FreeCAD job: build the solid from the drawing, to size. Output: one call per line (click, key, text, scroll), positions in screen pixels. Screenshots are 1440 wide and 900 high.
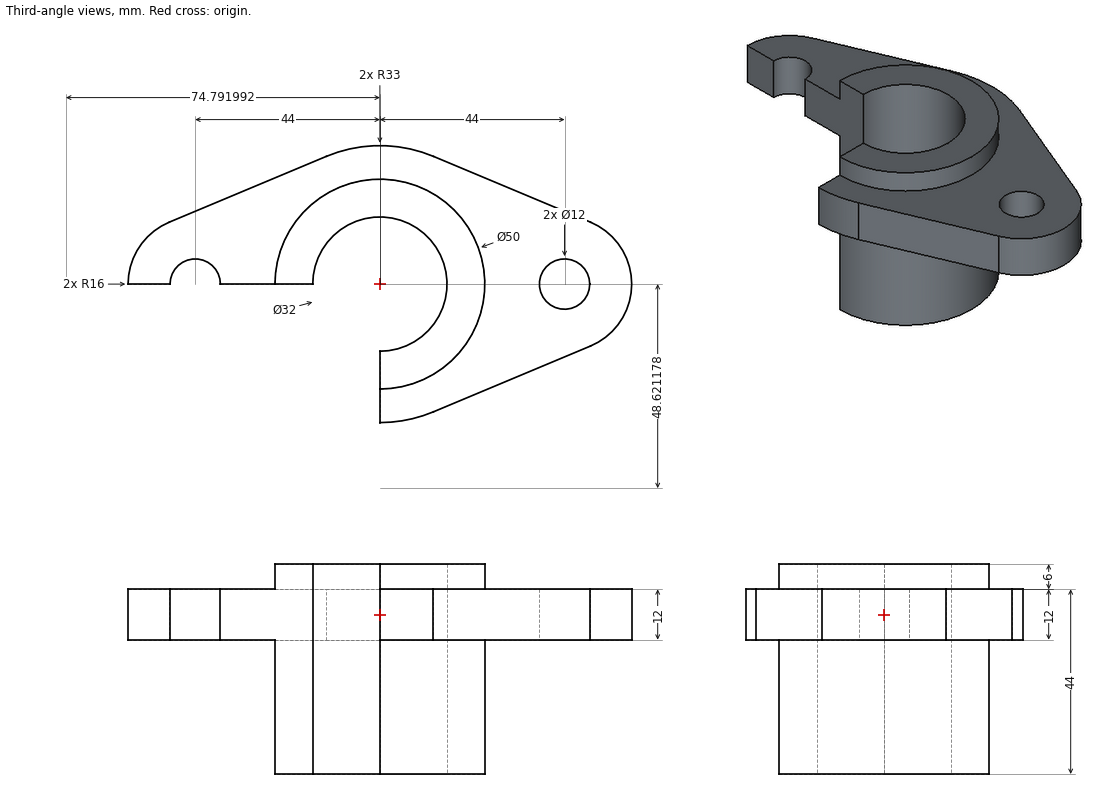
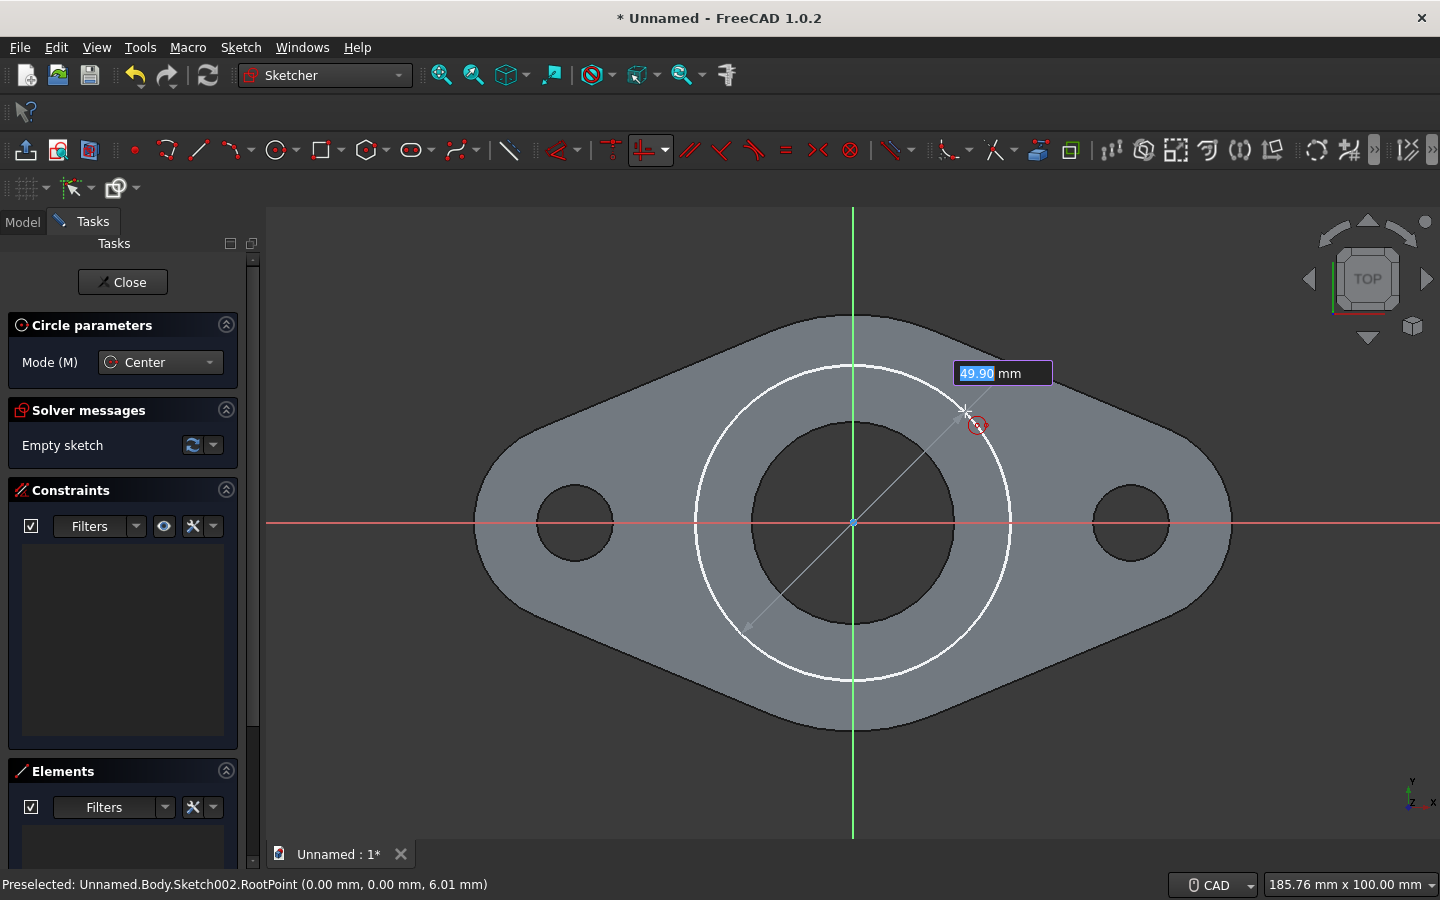
text(50)
key(Return)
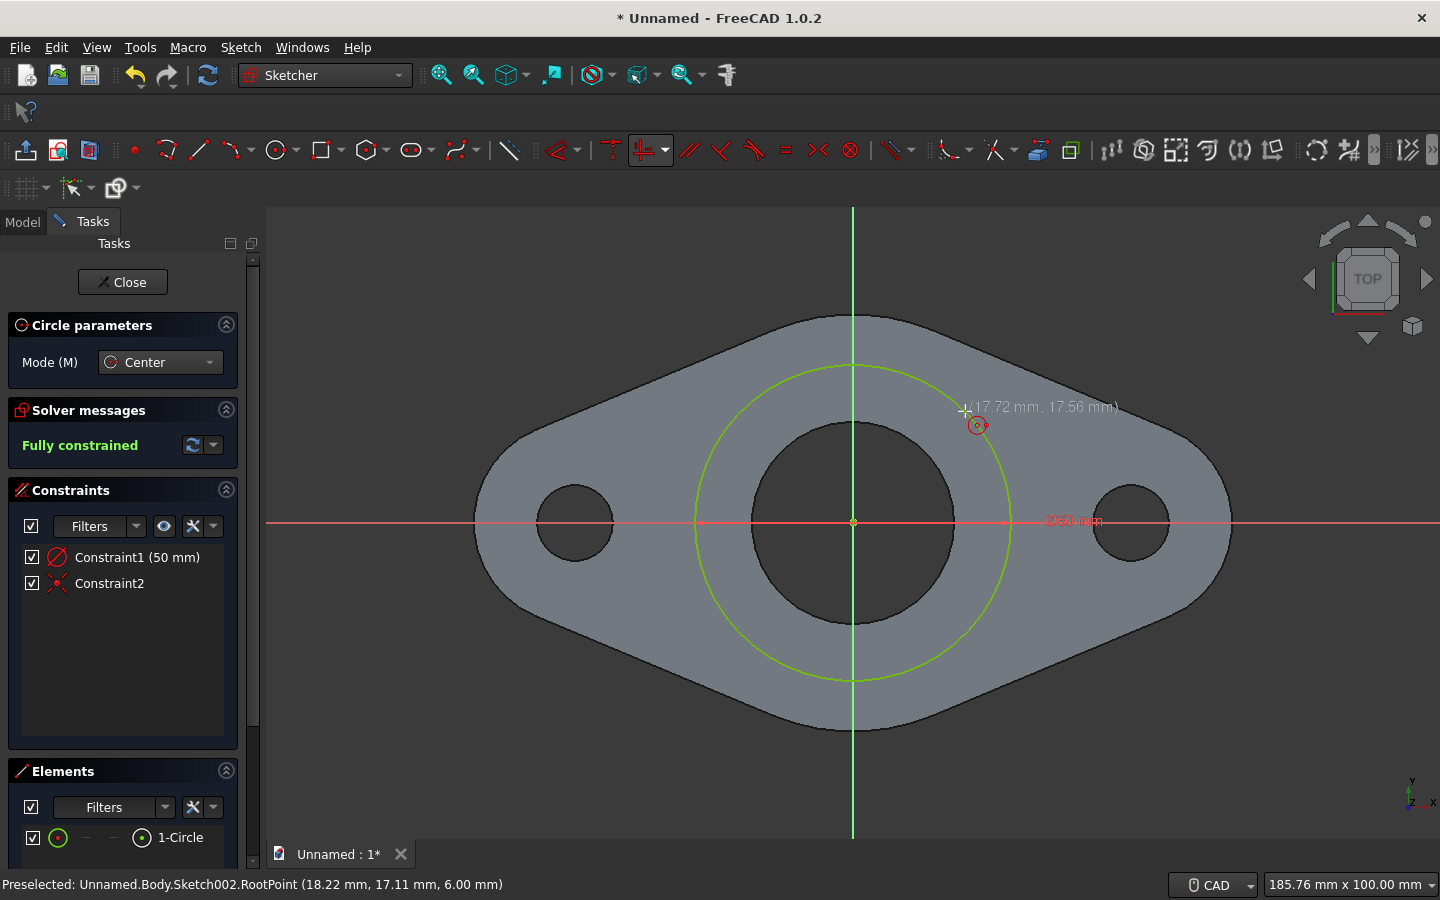
click(853, 523)
move(925, 451)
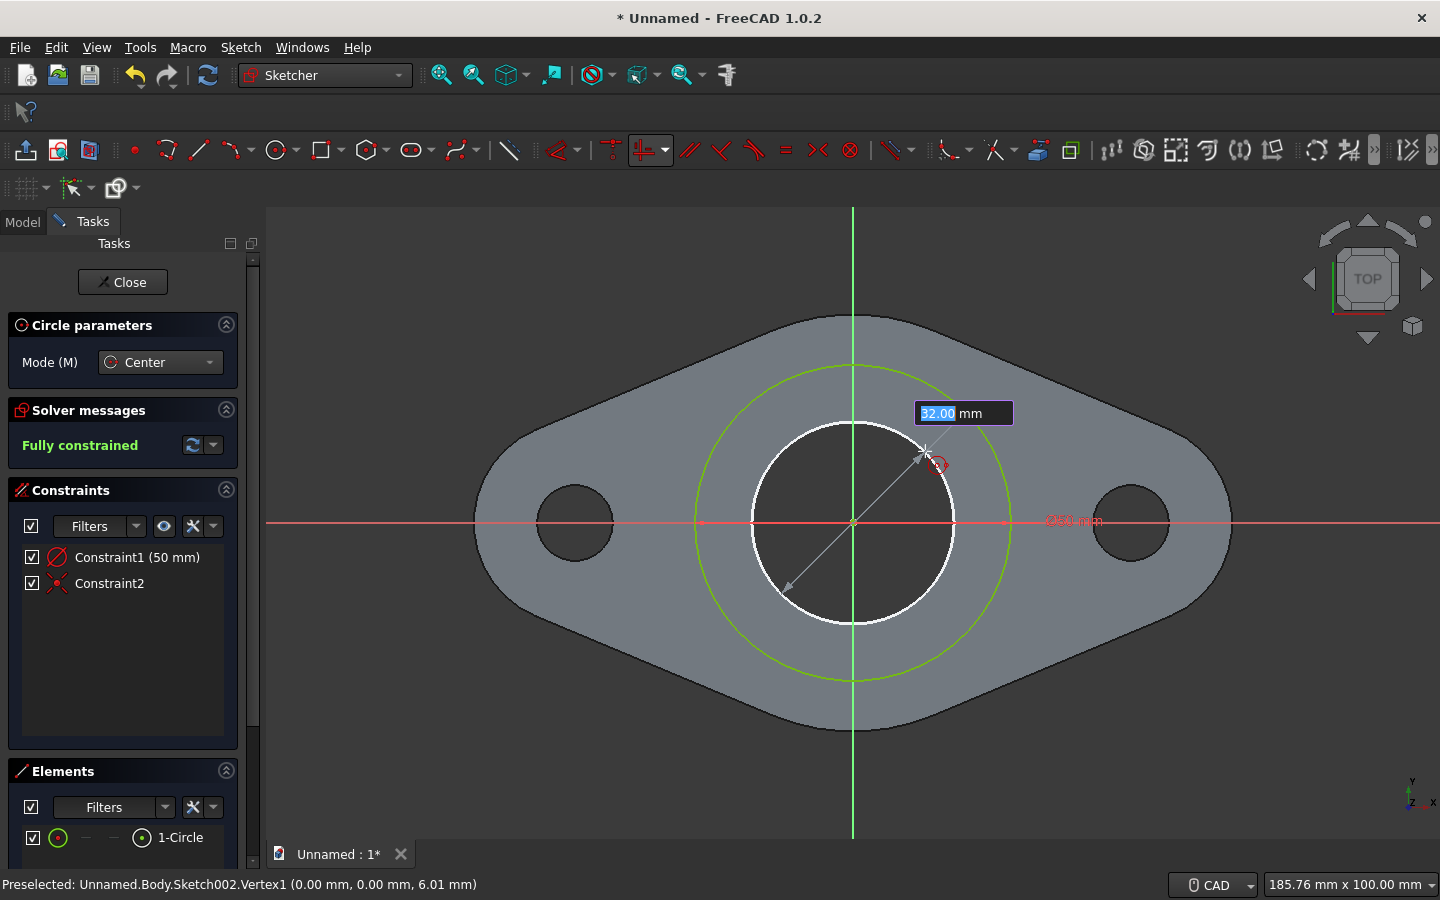
text(32)
key(Return)
key(Escape)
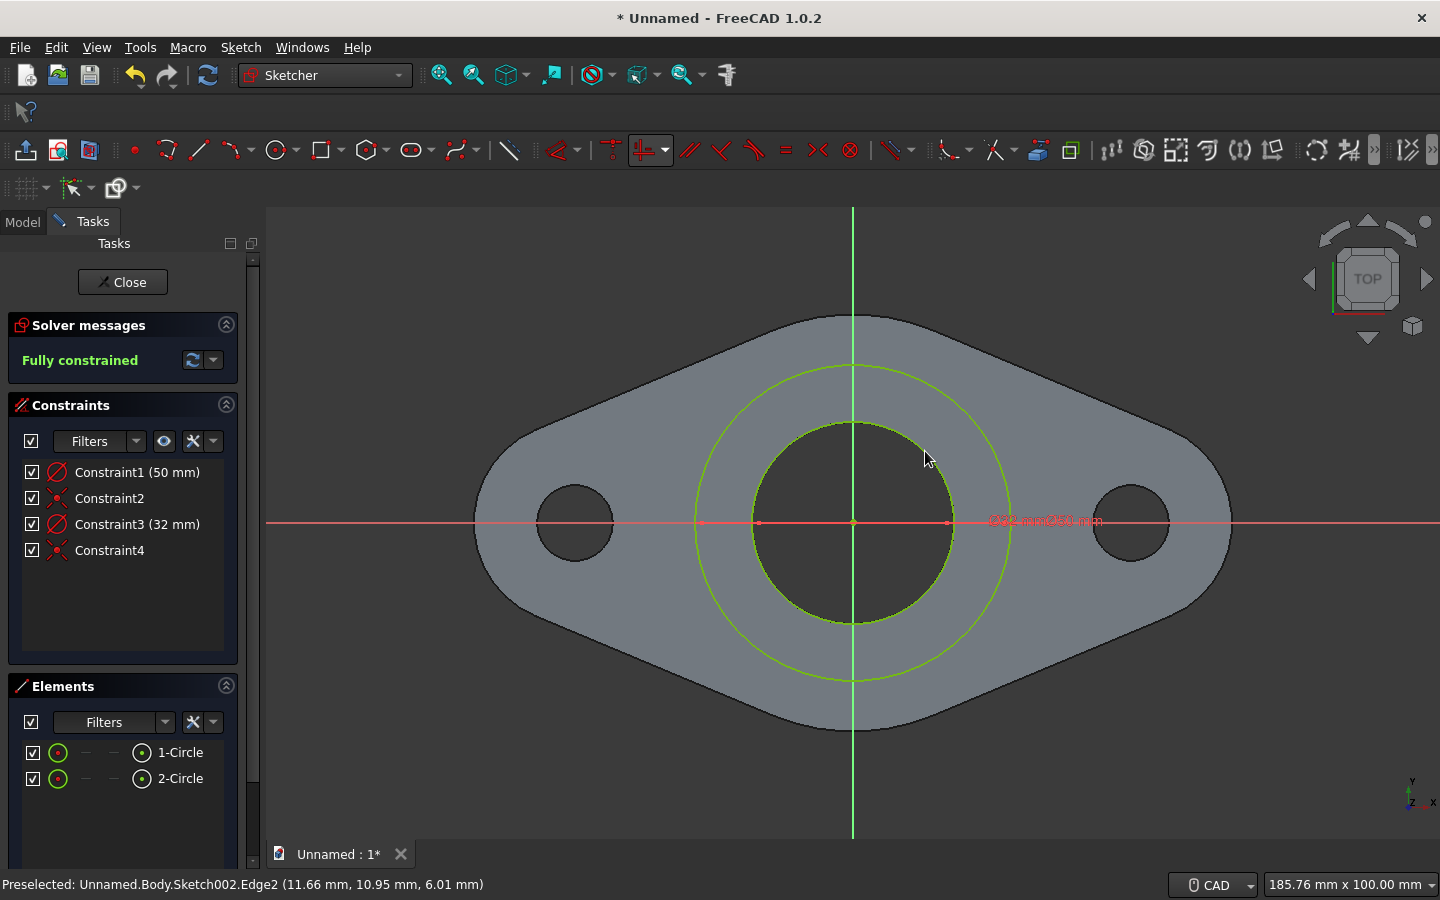
click(123, 282)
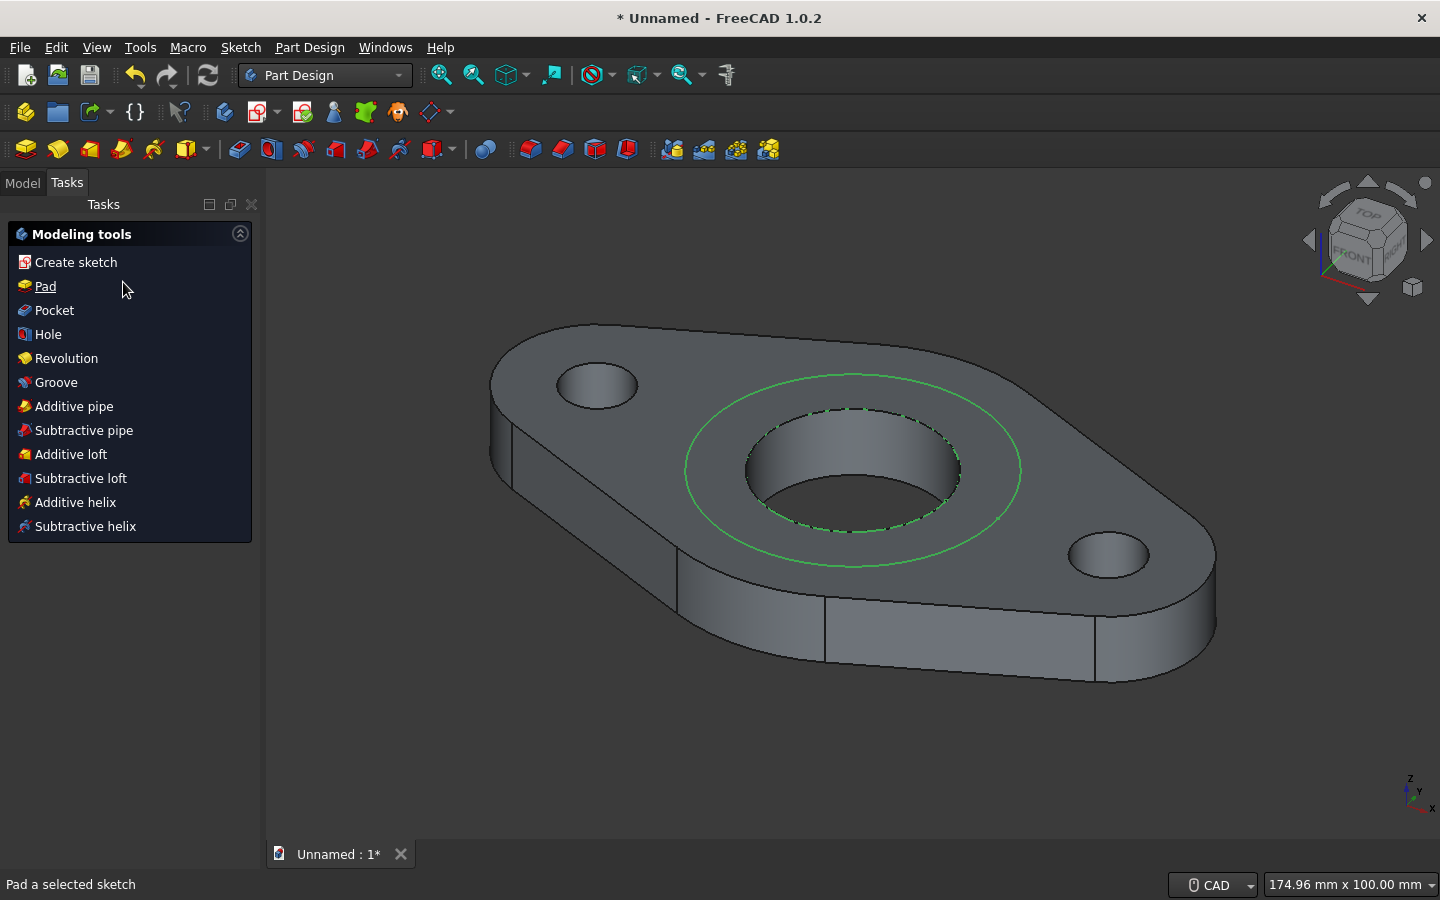
click(26, 150)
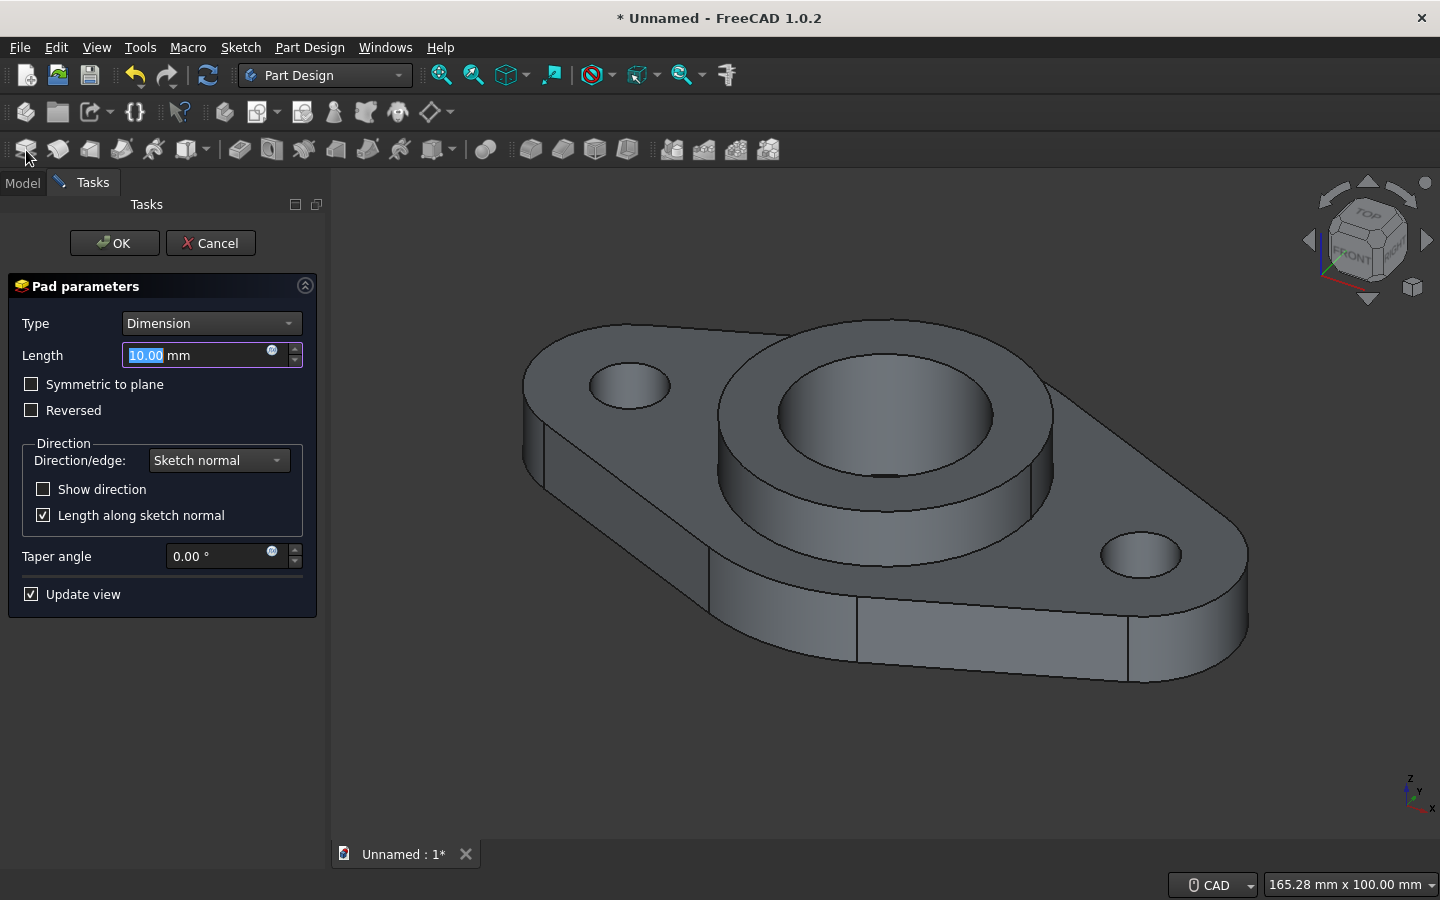
click(212, 324)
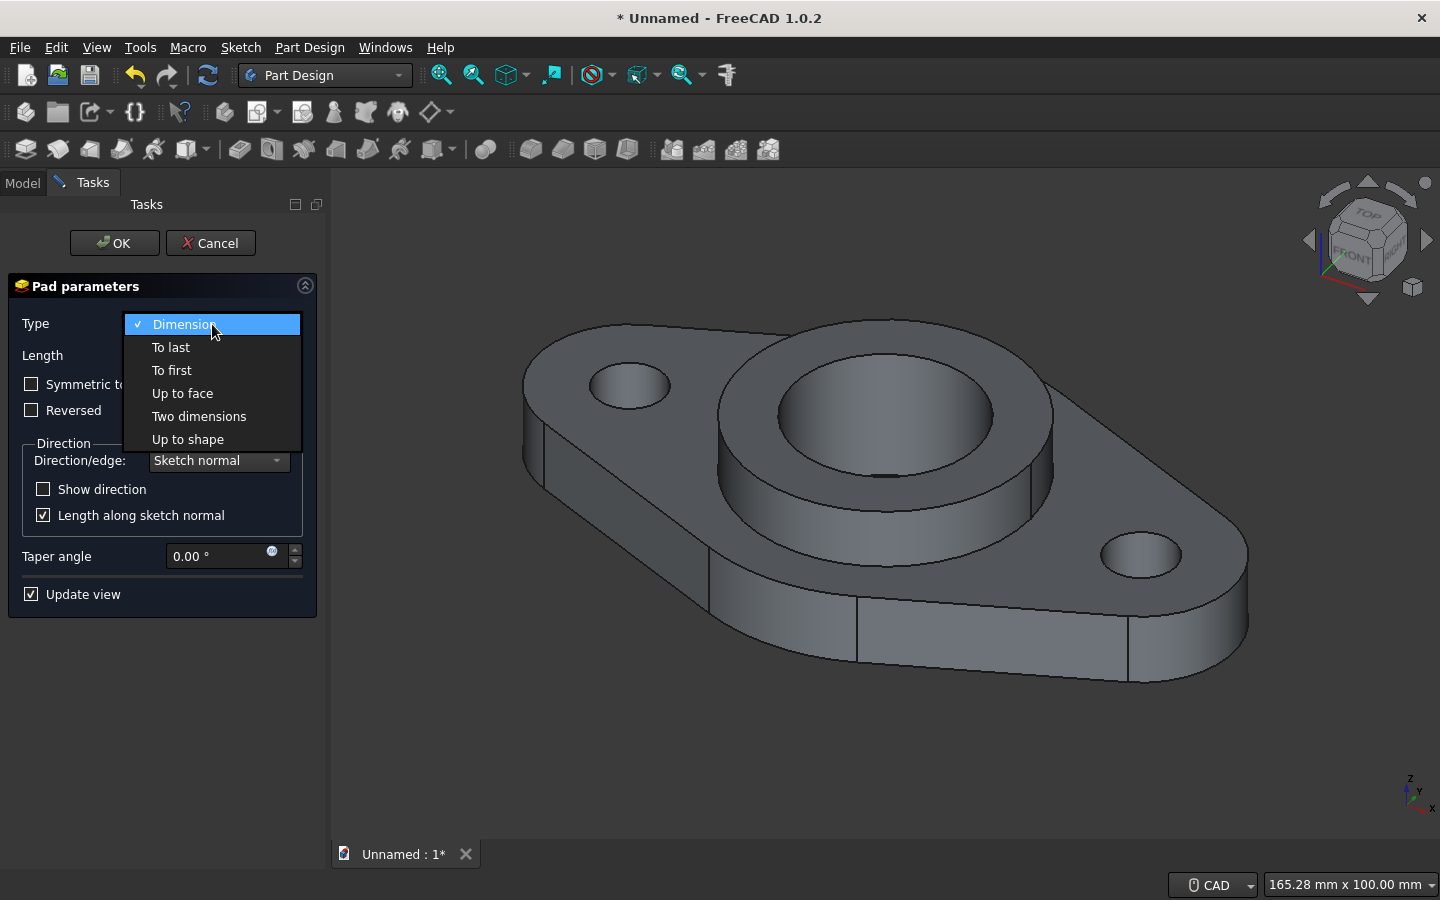
click(212, 416)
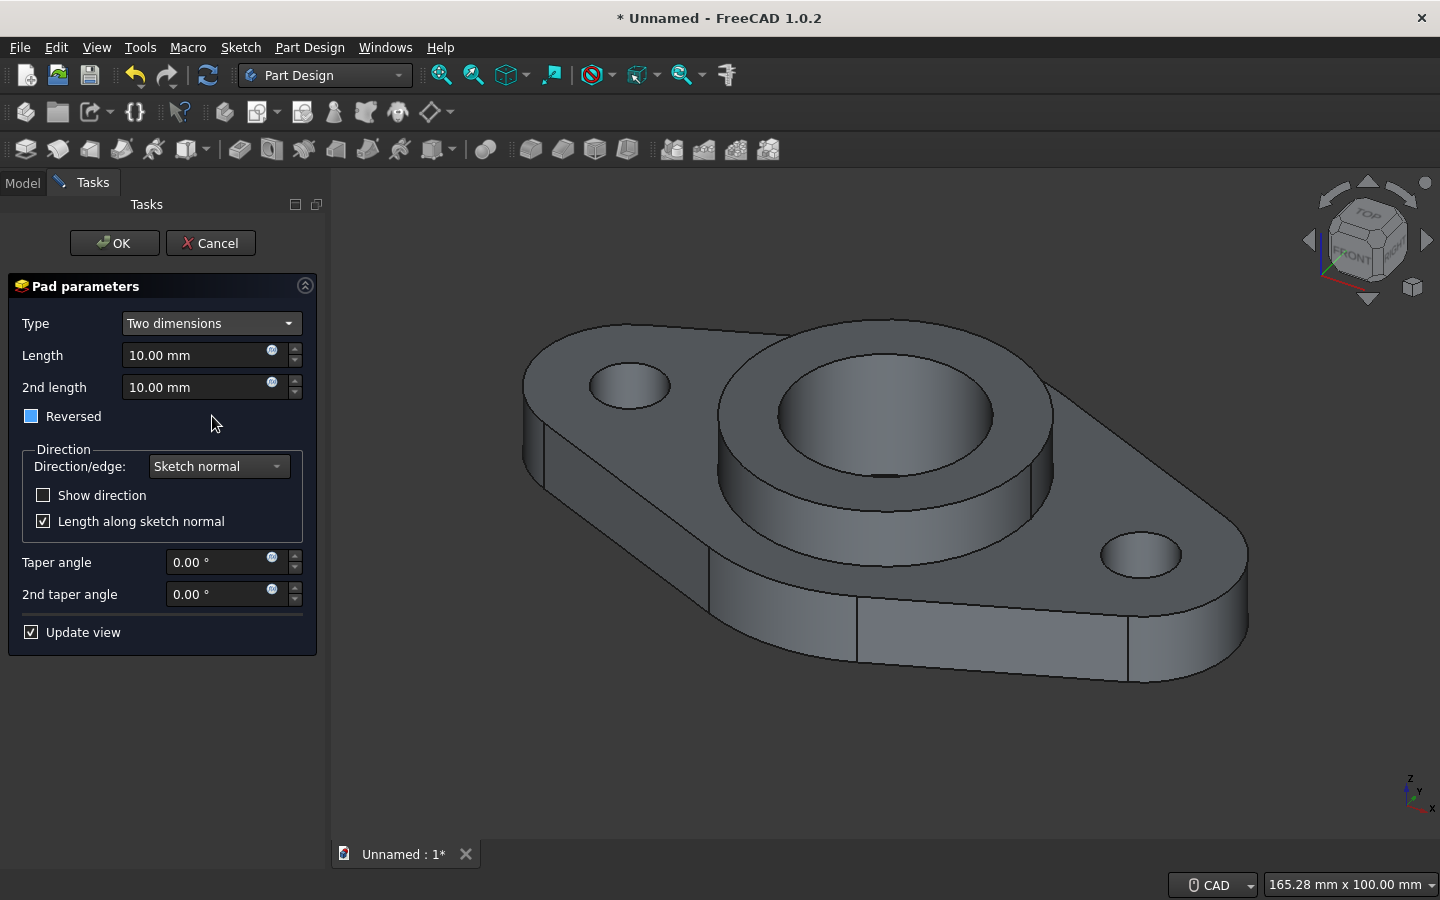
triple_click(204, 355)